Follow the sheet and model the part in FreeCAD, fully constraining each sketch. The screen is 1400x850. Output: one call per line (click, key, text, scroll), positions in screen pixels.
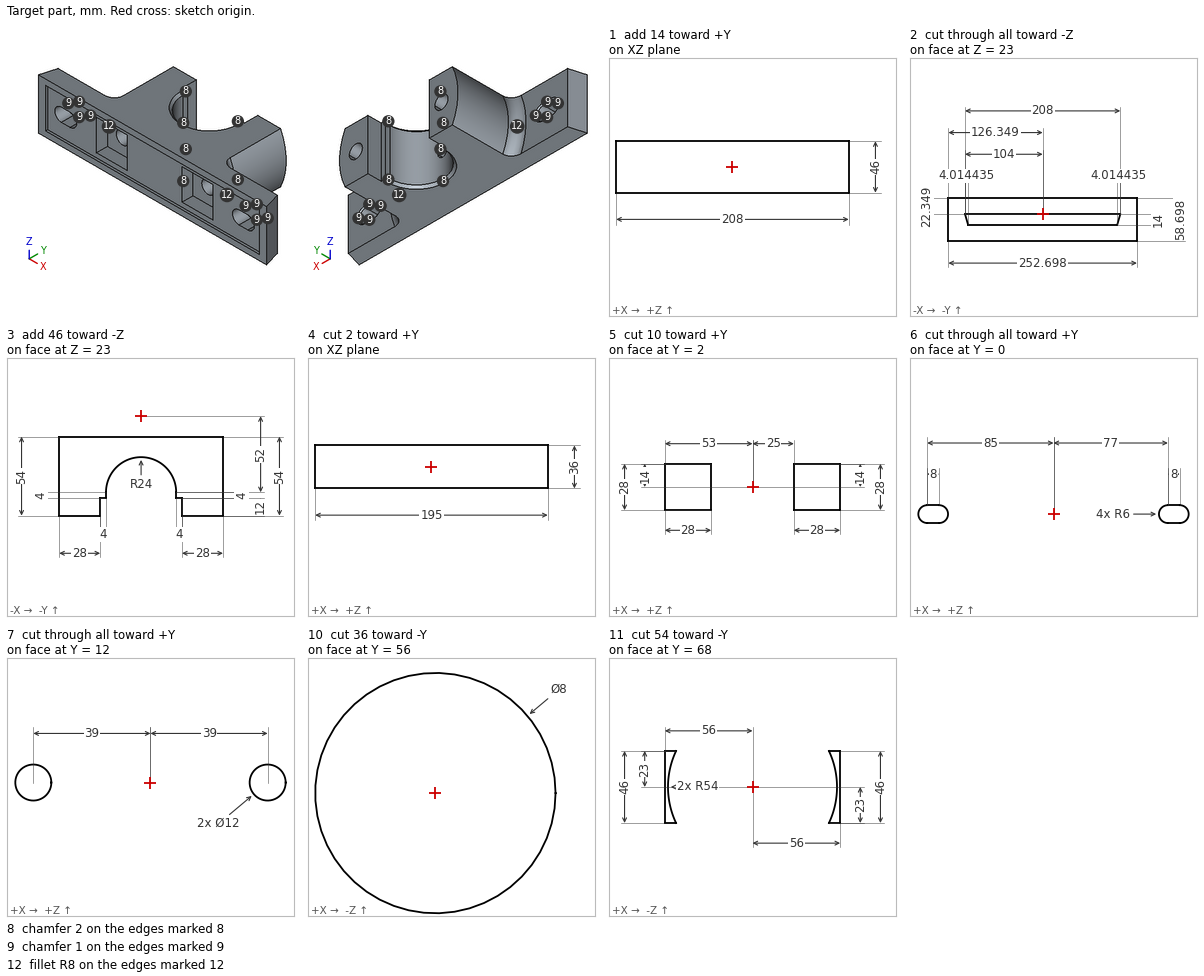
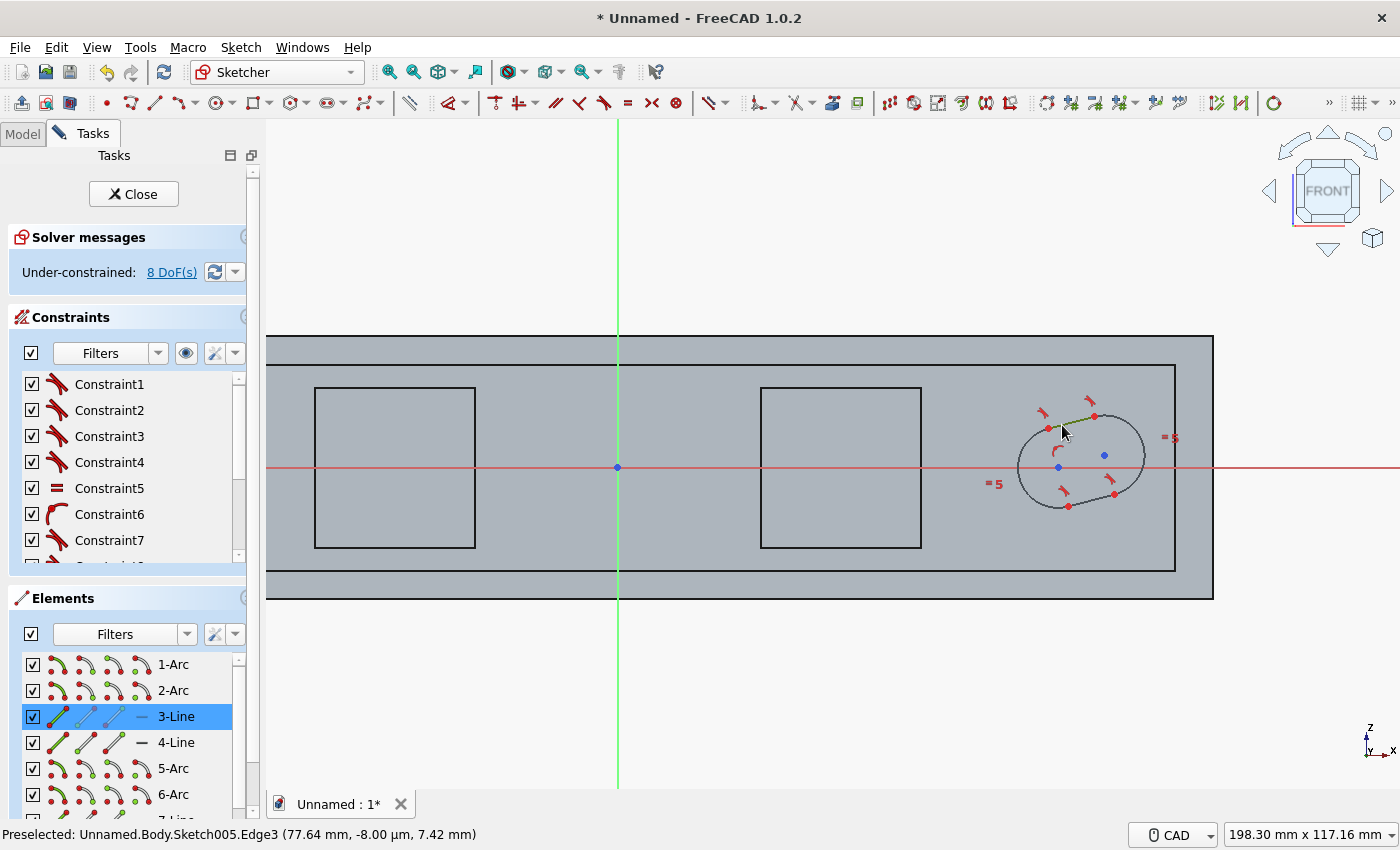
click(538, 104)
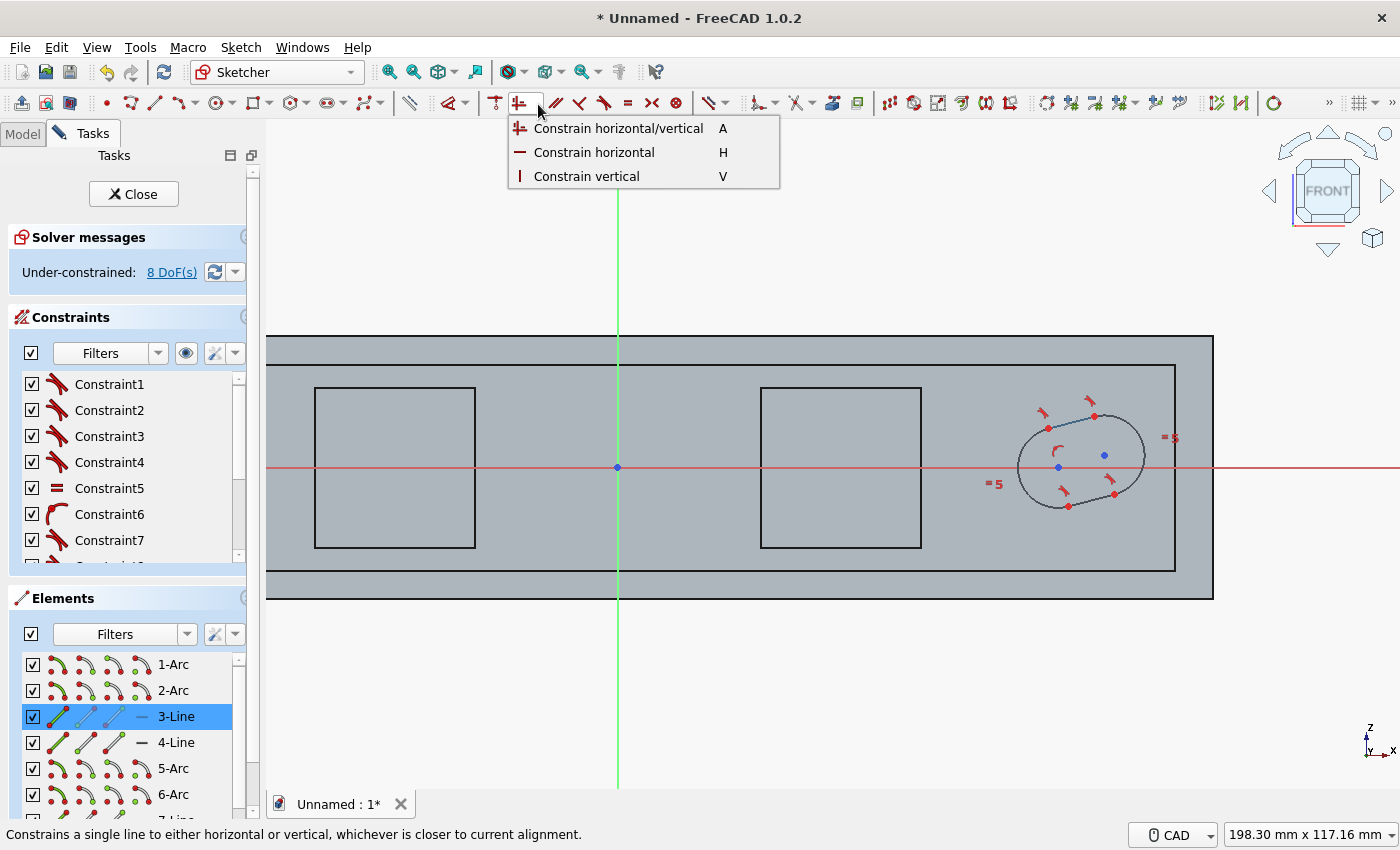
click(644, 152)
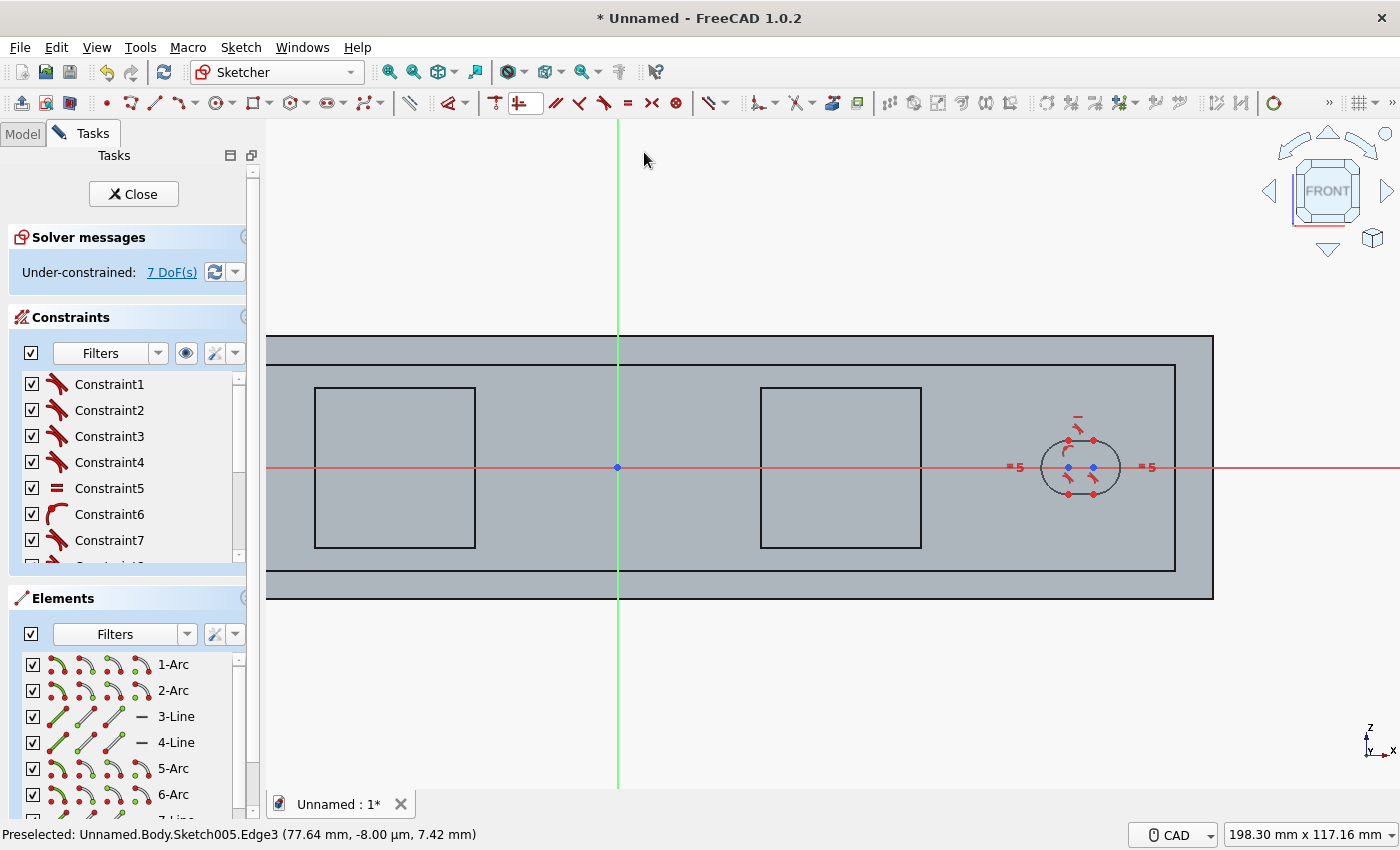
scroll(1063, 426, down, 2)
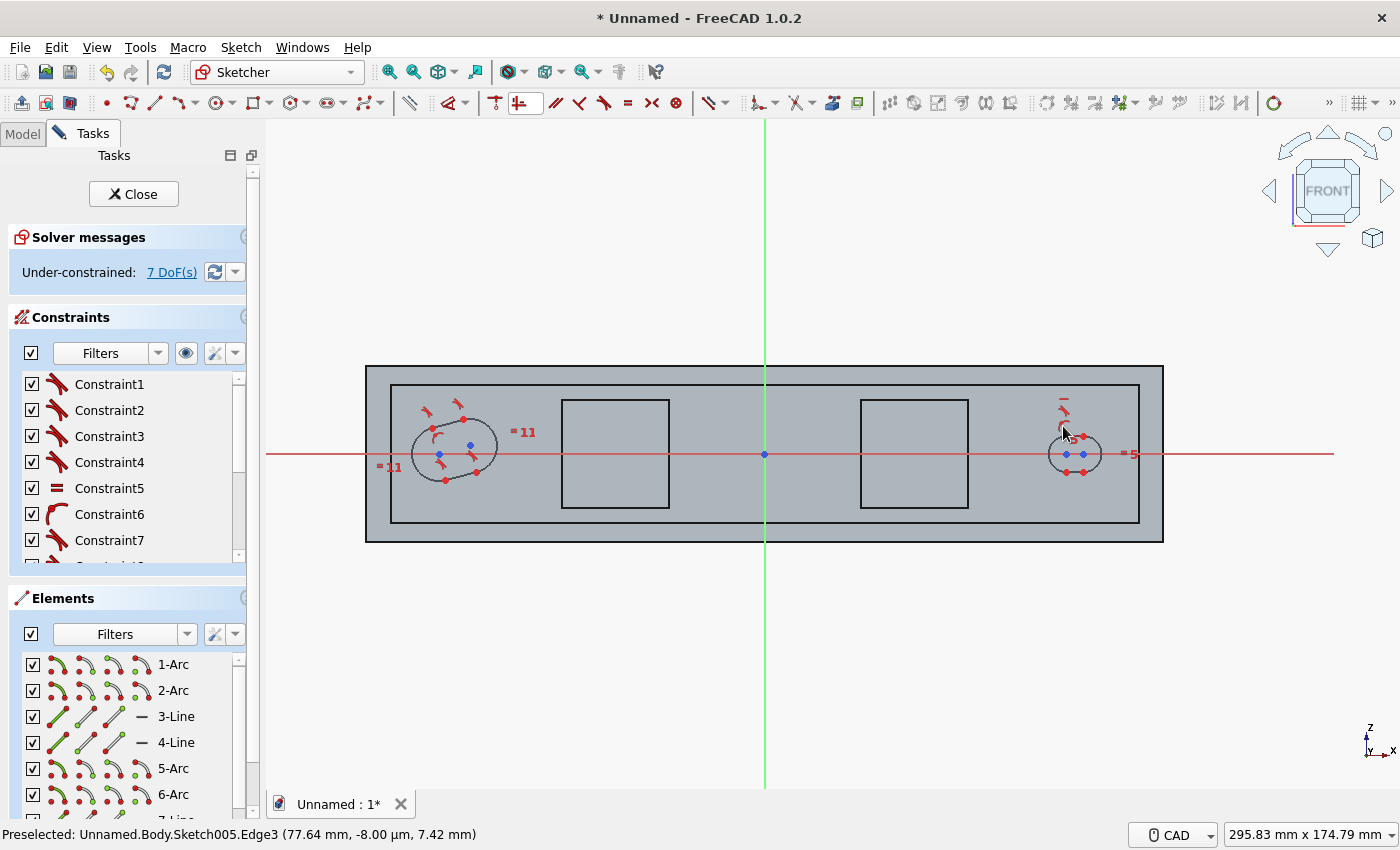
scroll(442, 426, up, 2)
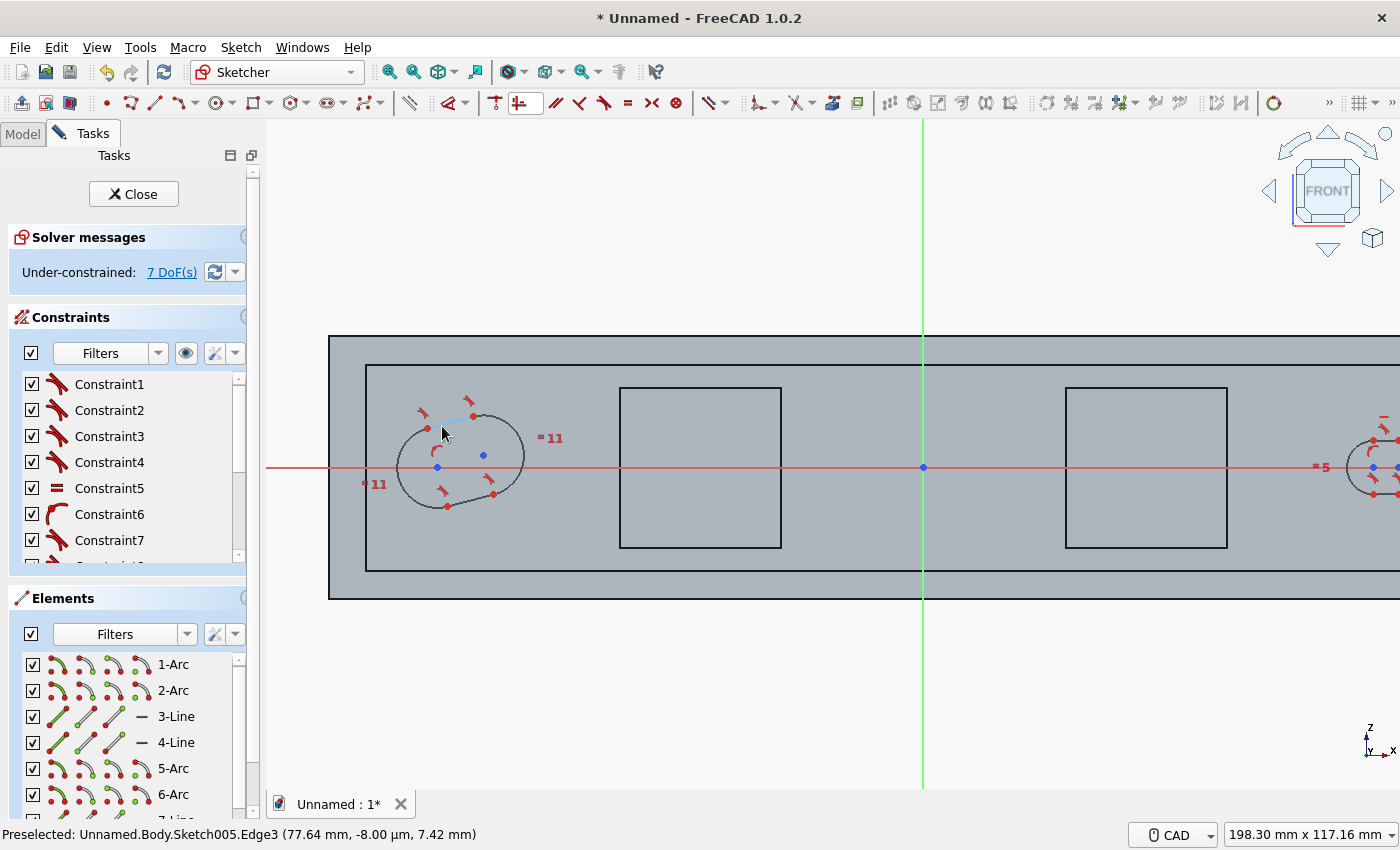
click(441, 425)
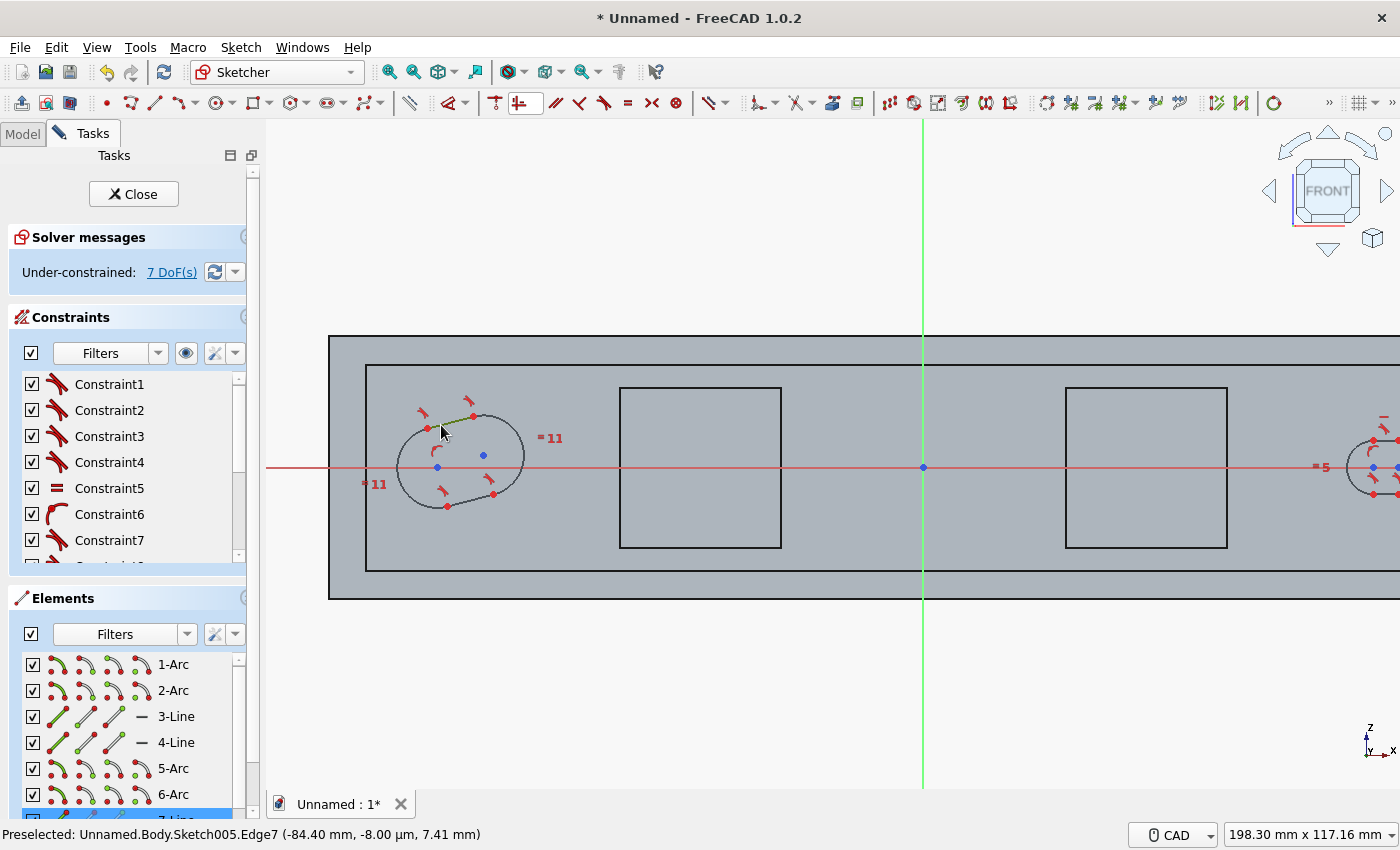
key(h)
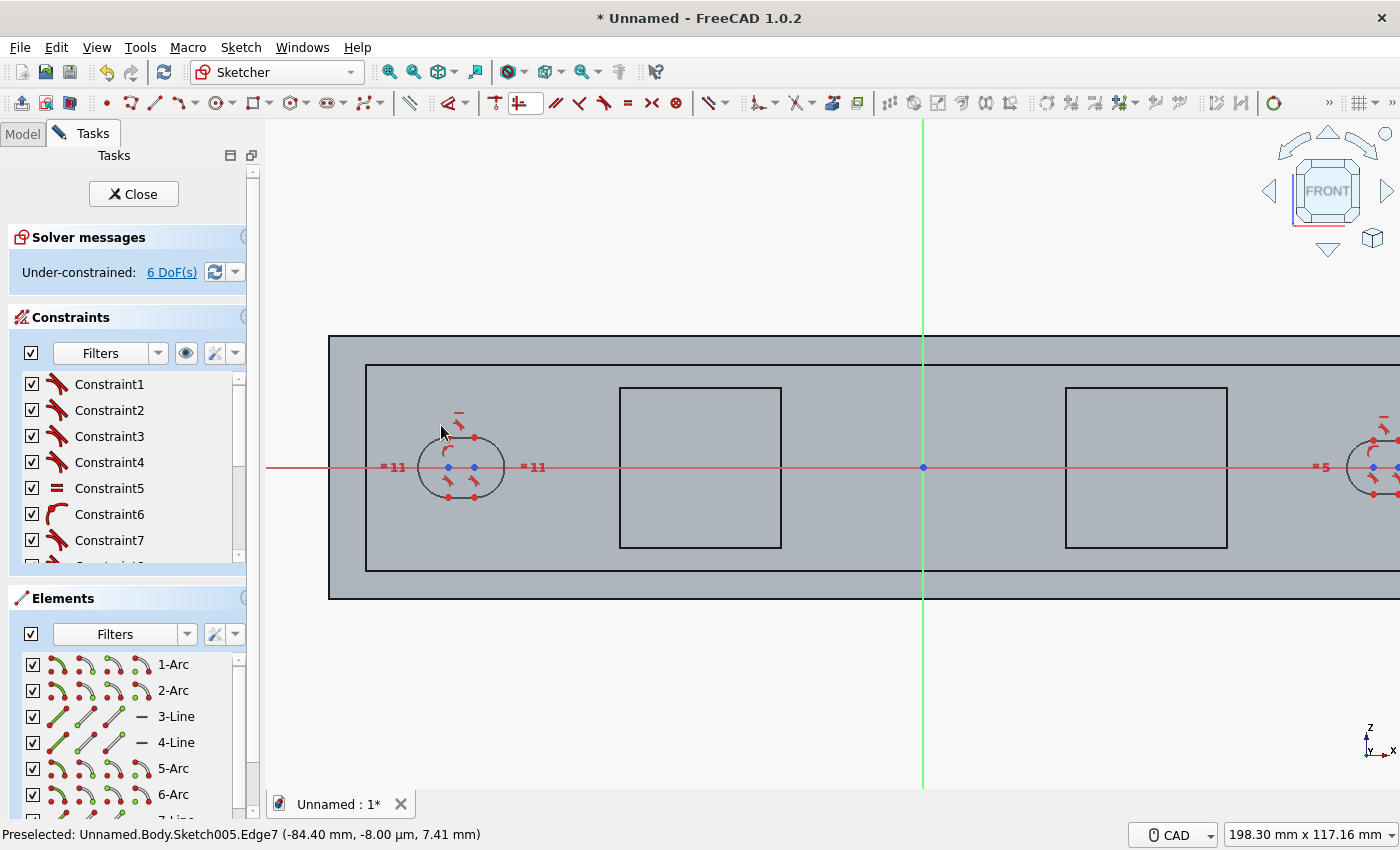
scroll(441, 426, down, 2)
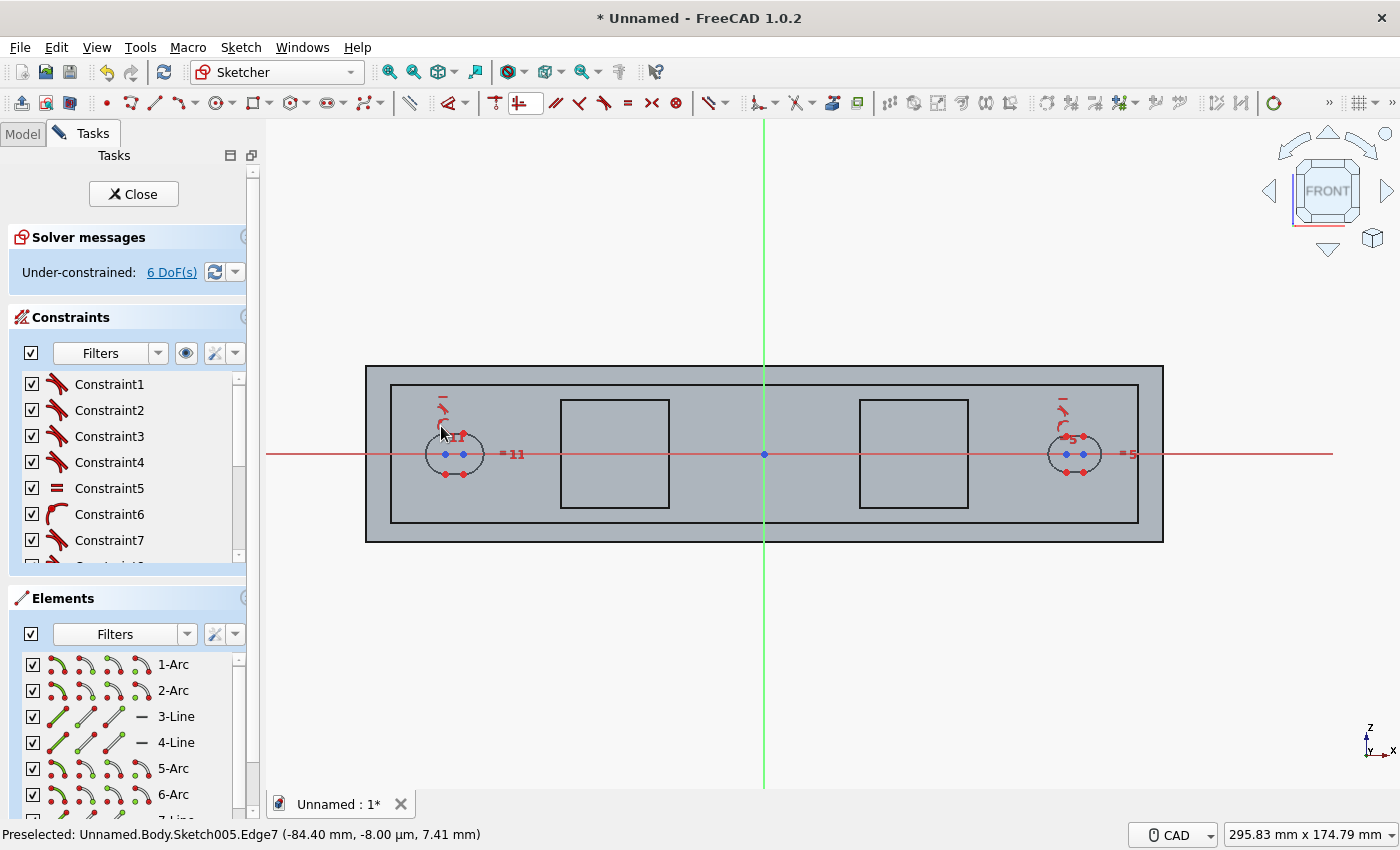
scroll(1052, 444, up, 2)